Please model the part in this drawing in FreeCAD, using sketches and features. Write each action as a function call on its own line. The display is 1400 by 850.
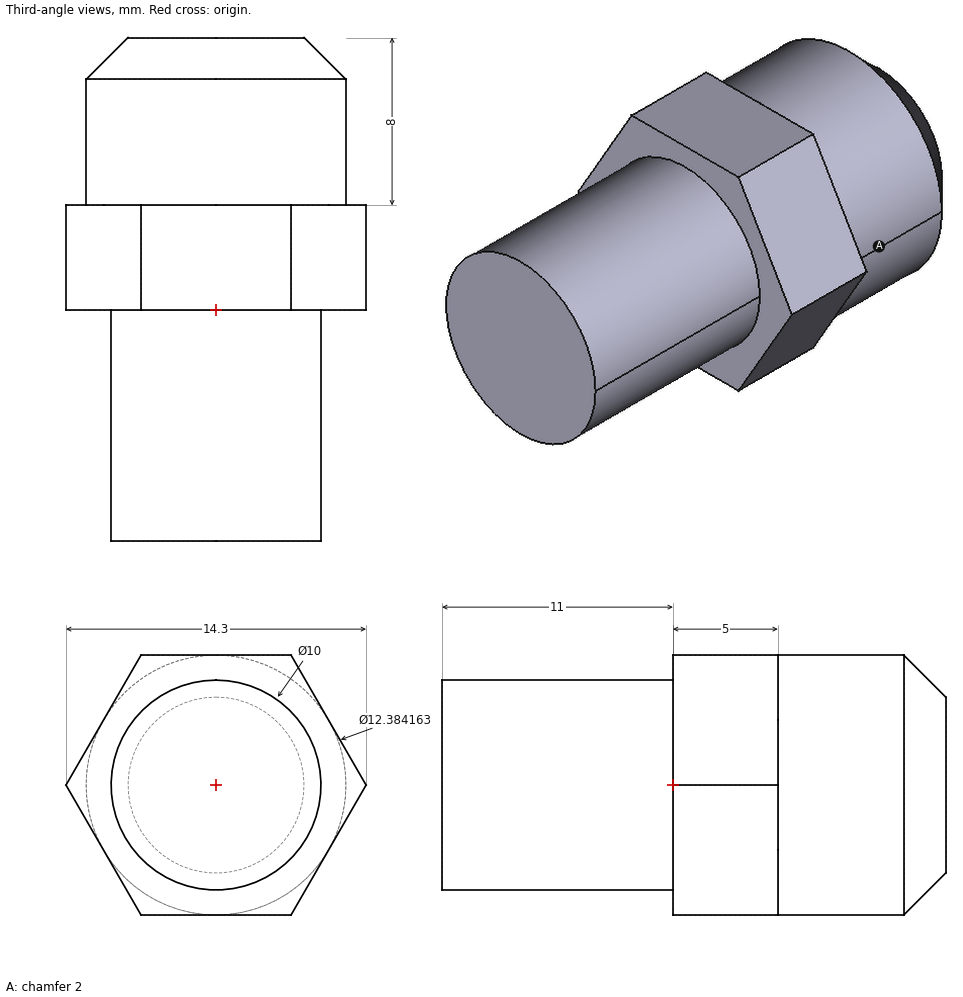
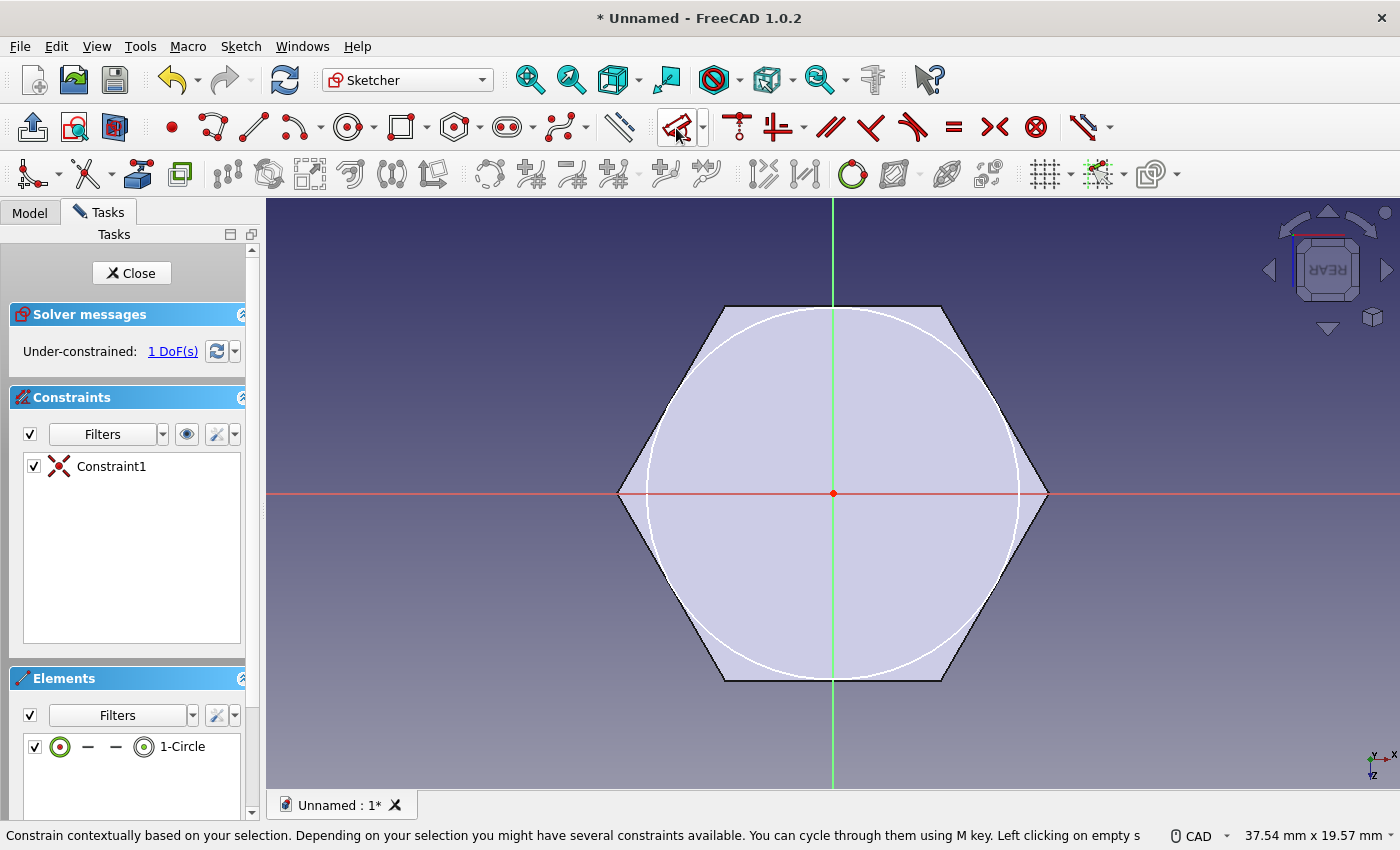
click(964, 361)
click(986, 338)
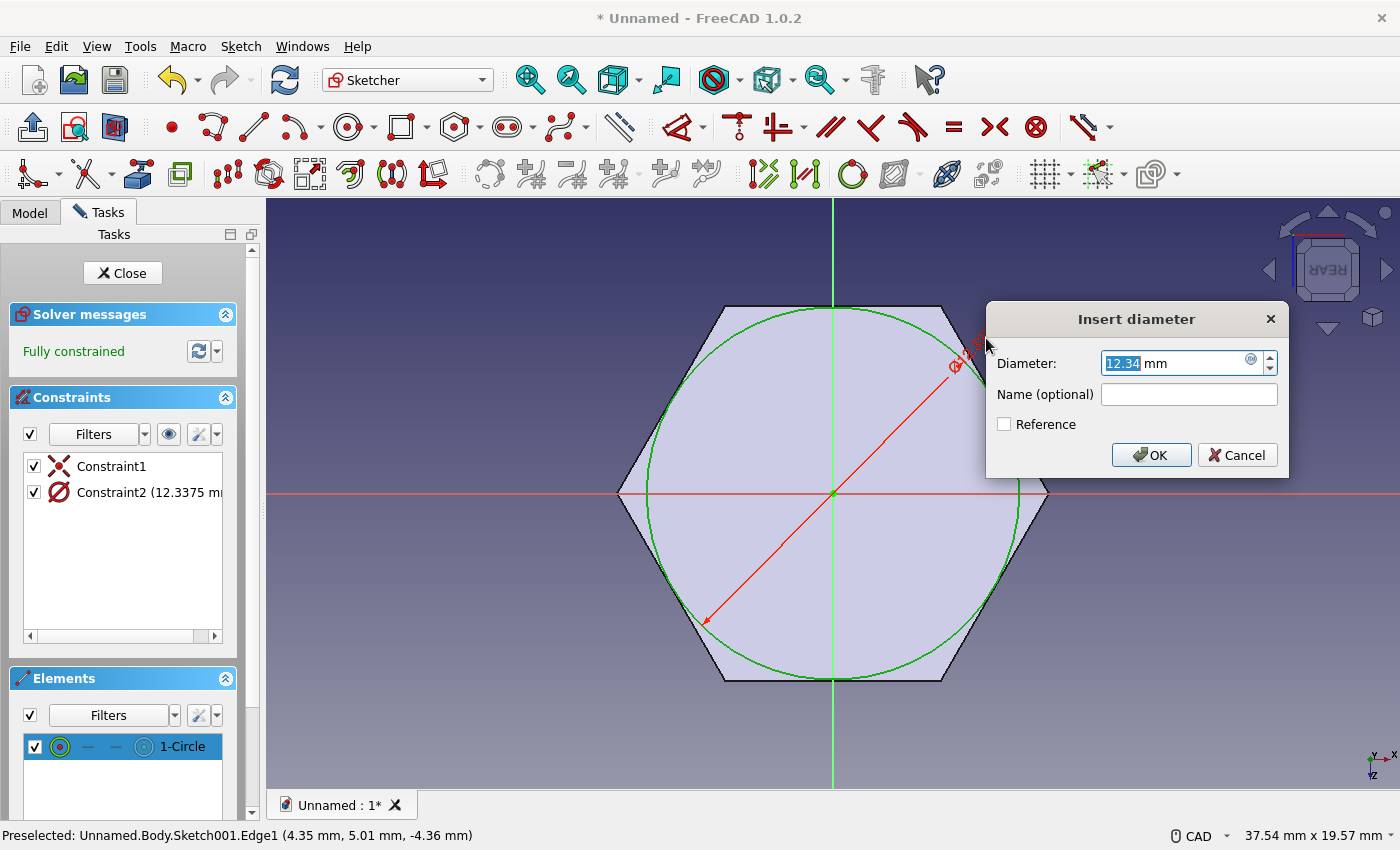
text(12.384163)
key(Return)
key(Escape)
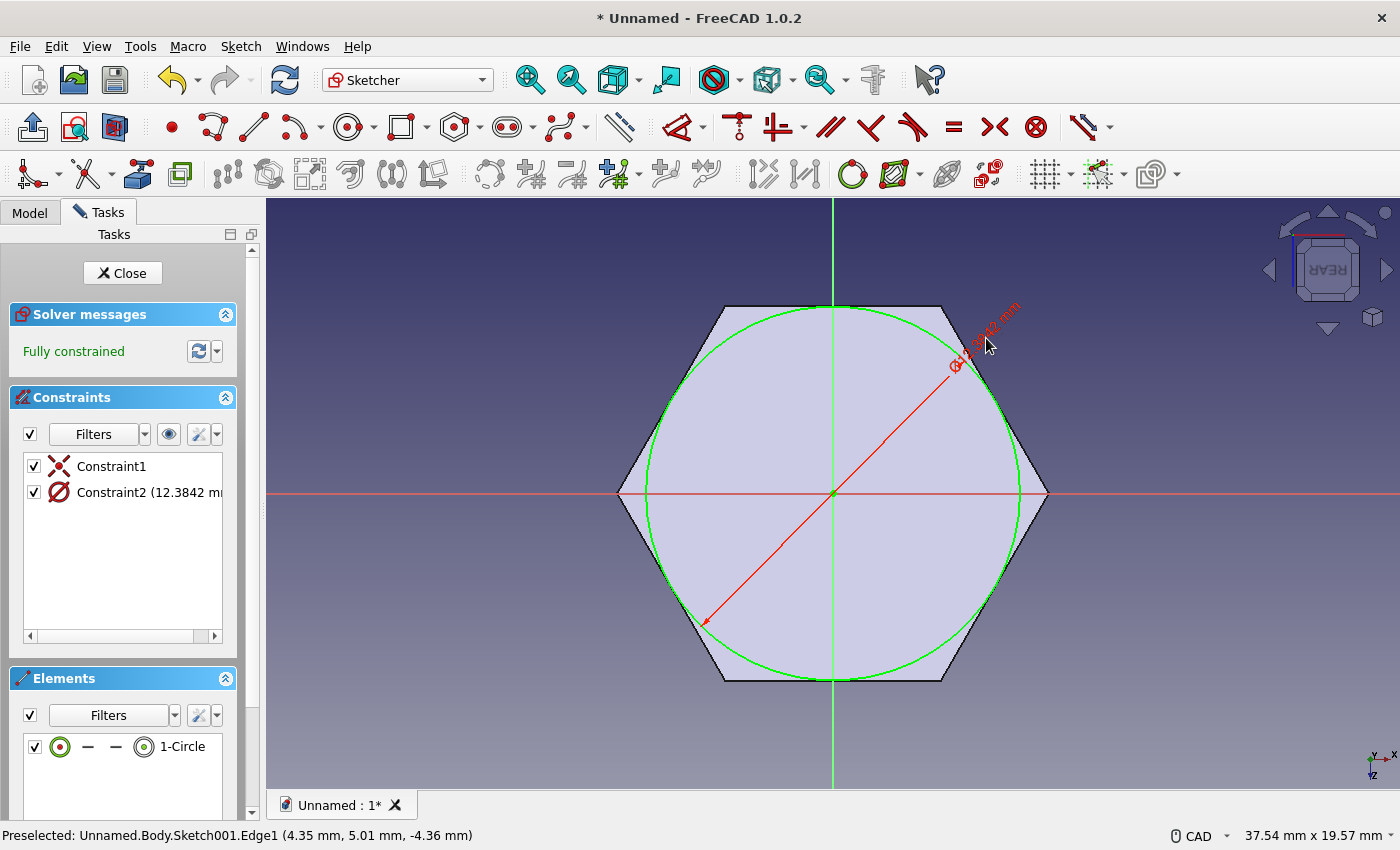
click(123, 273)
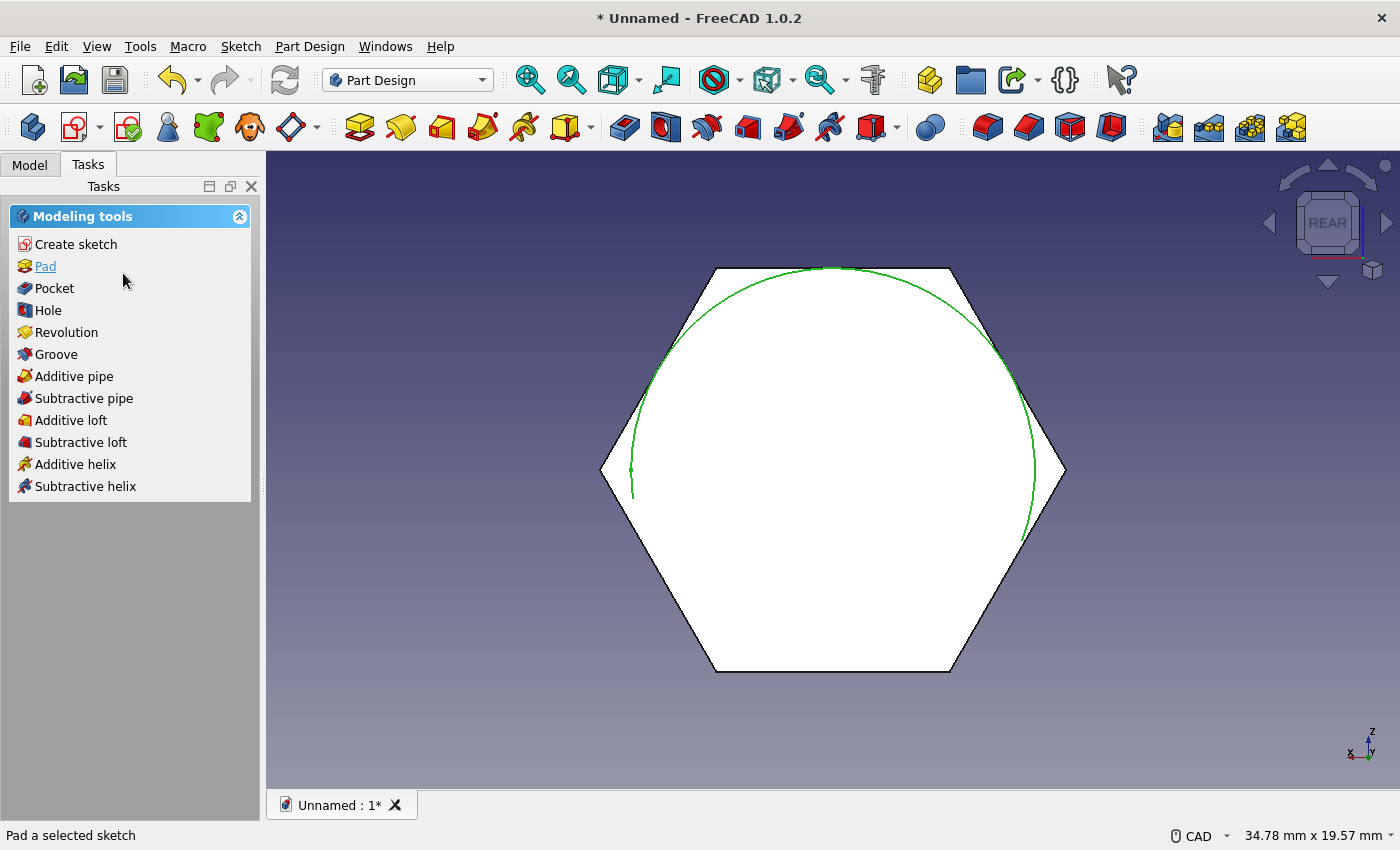
click(360, 128)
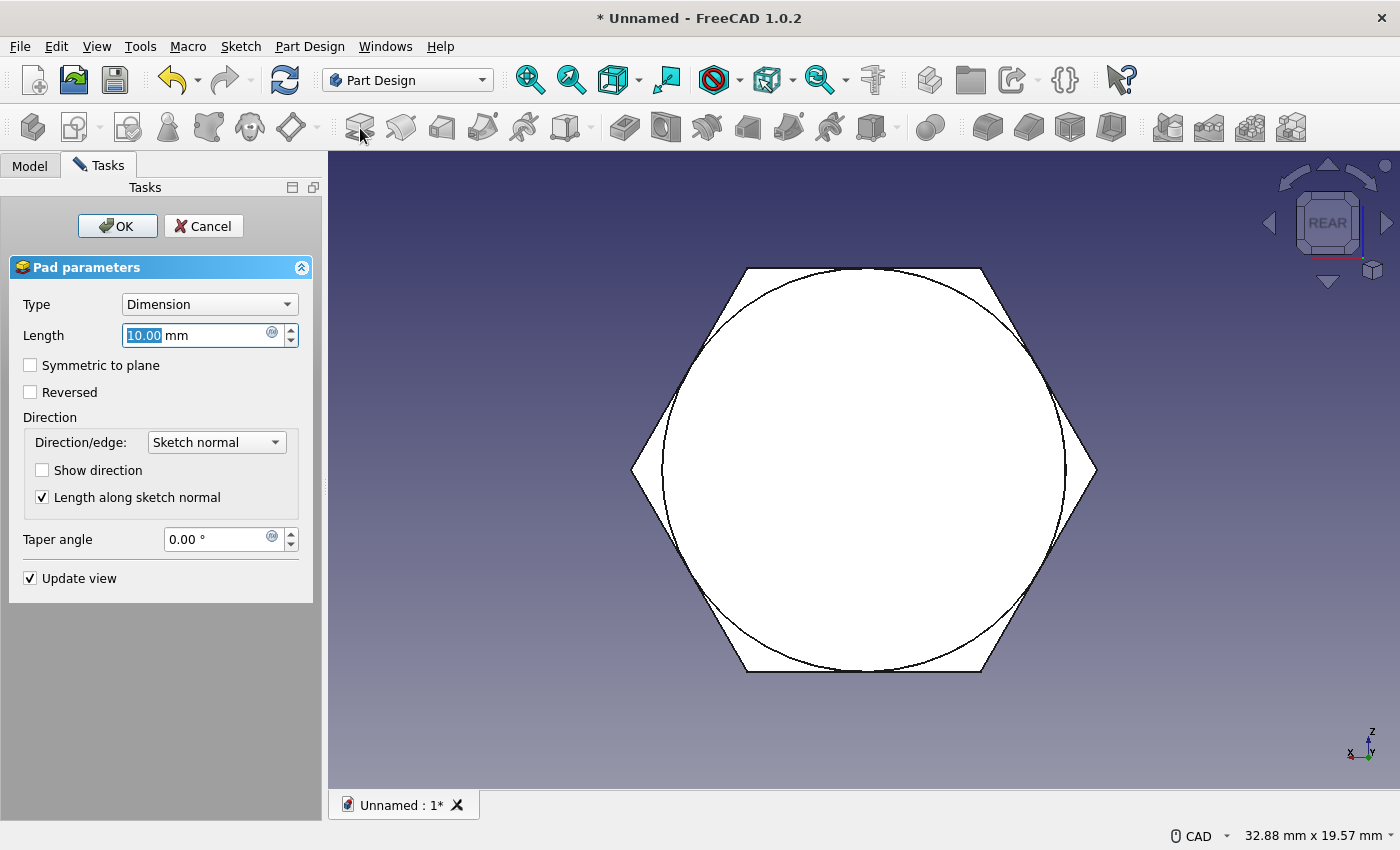
text(8)
key(Tab)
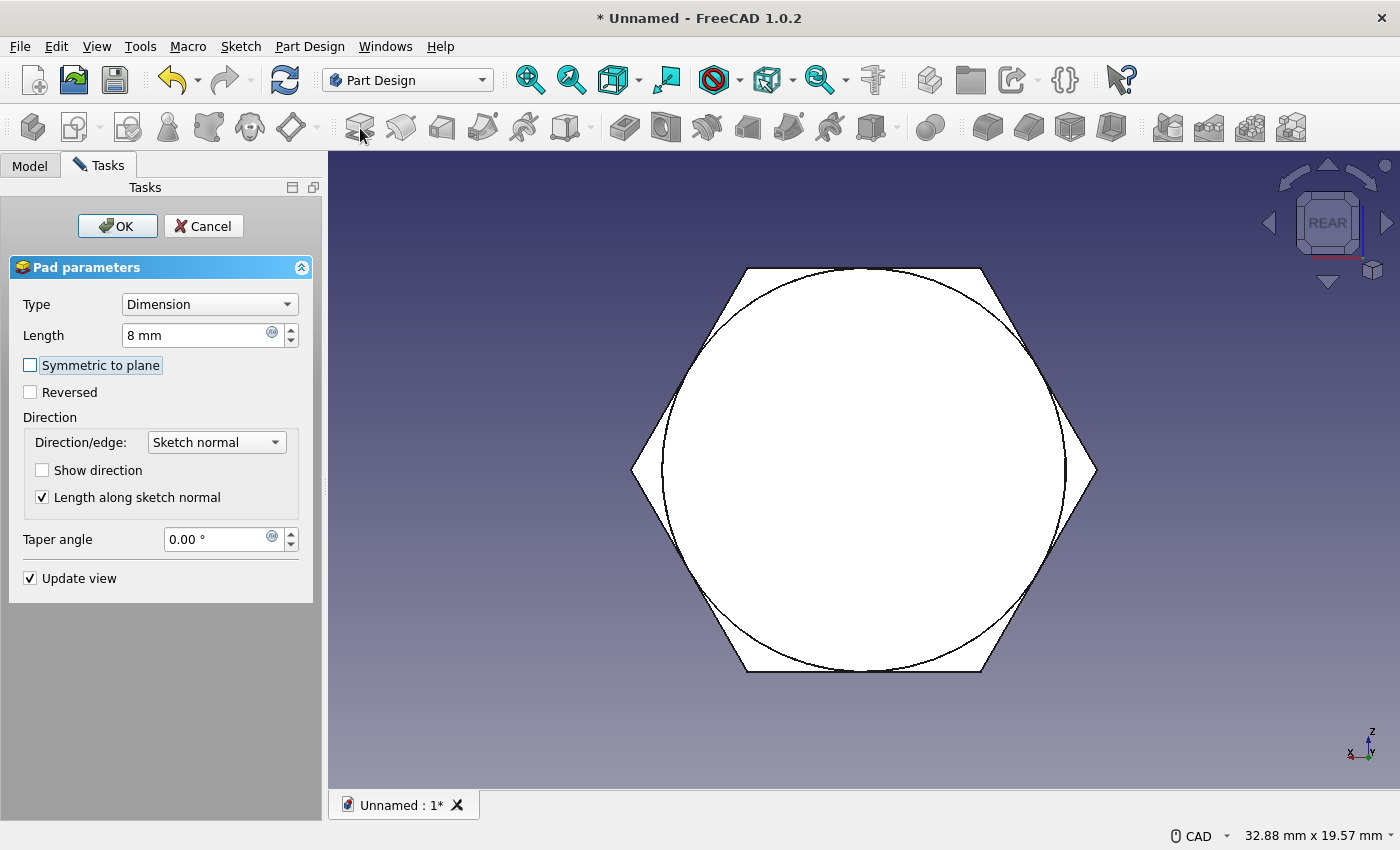
click(118, 226)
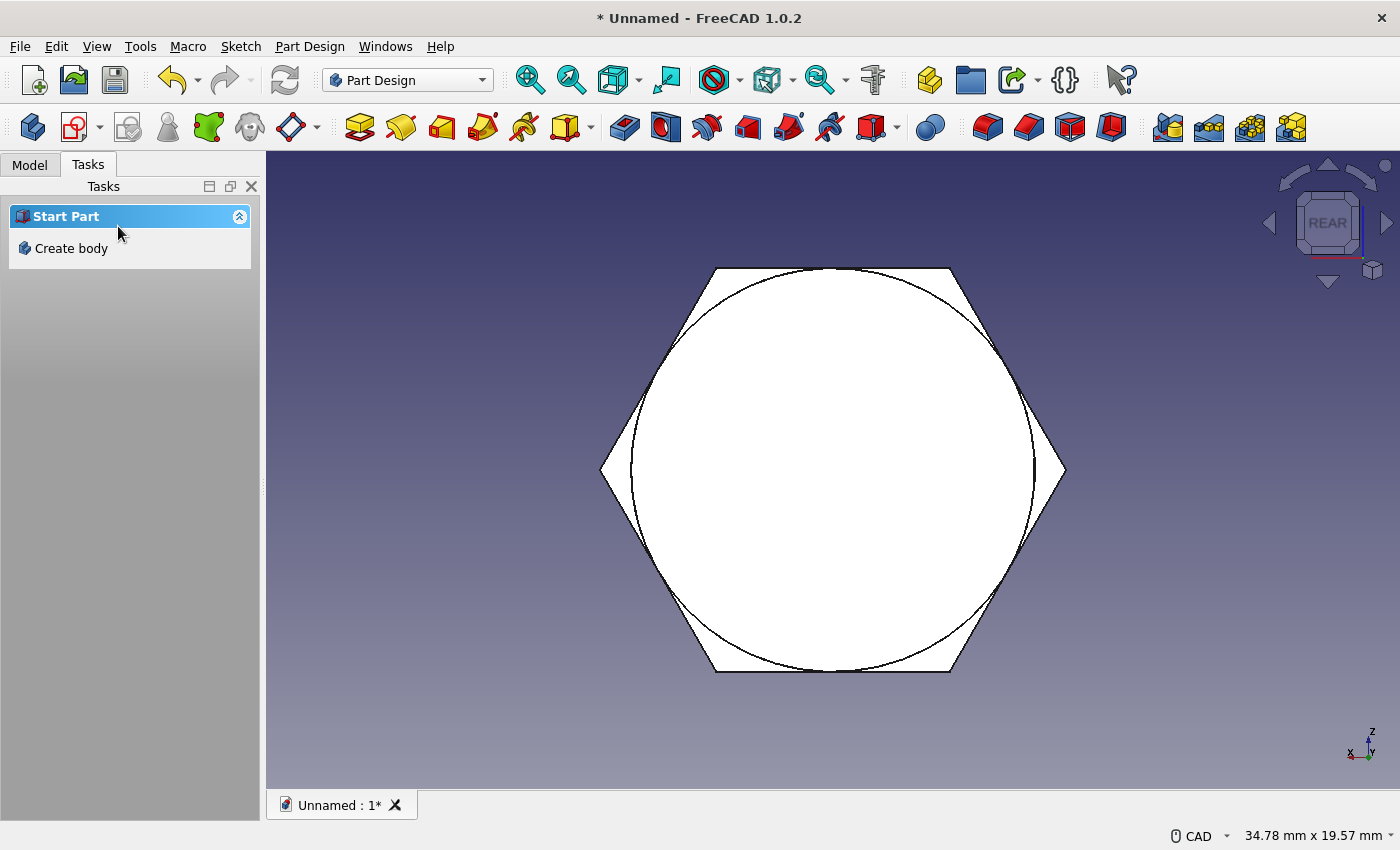
click(1035, 469)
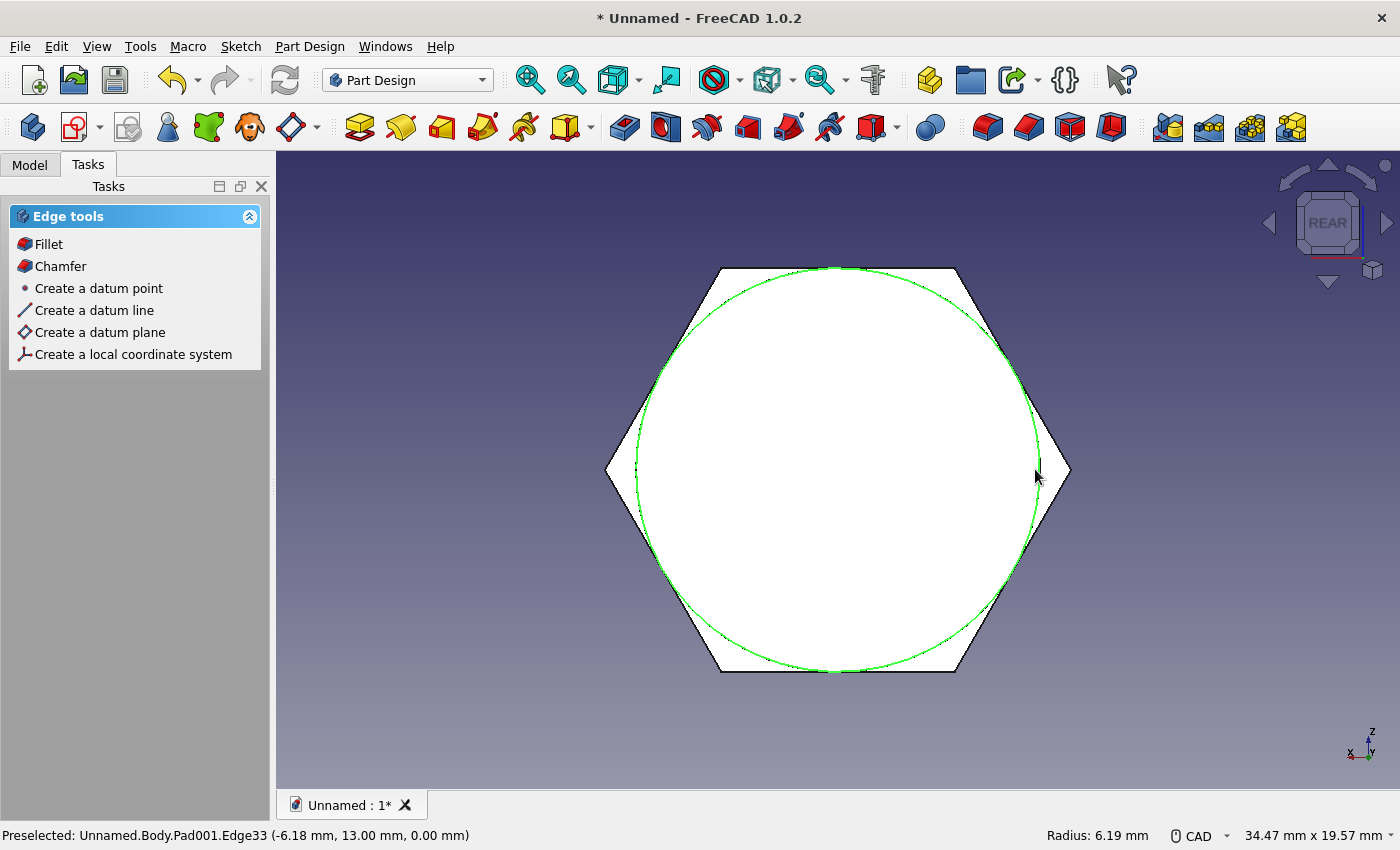
click(1029, 128)